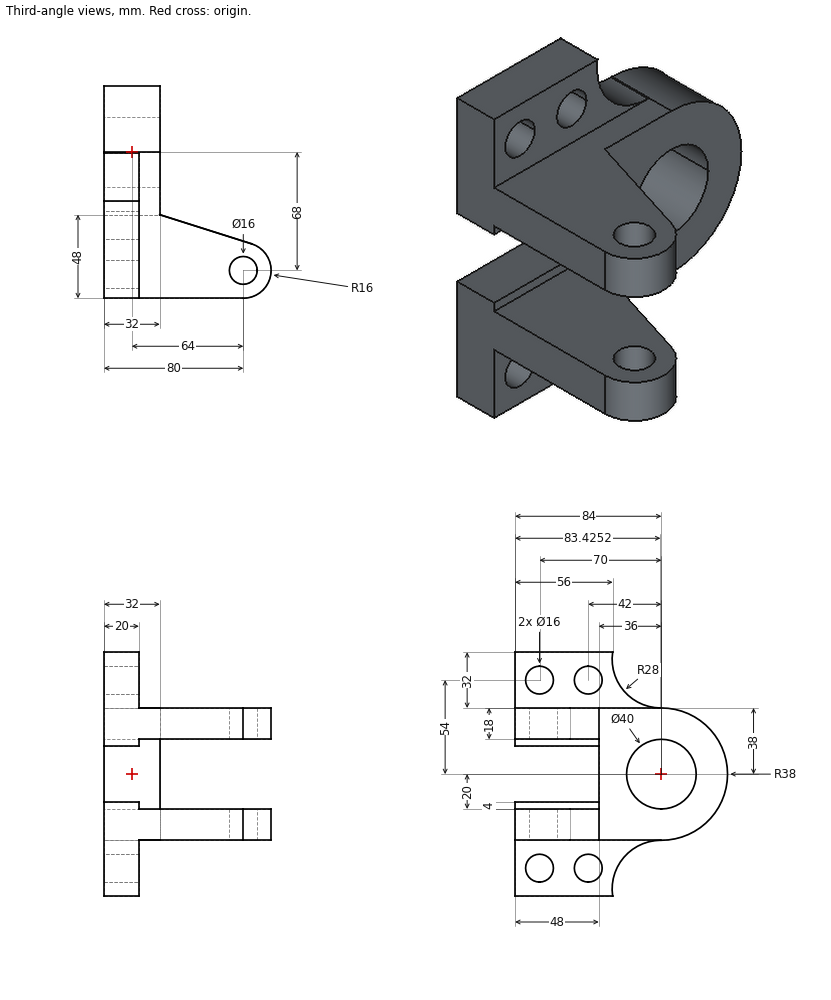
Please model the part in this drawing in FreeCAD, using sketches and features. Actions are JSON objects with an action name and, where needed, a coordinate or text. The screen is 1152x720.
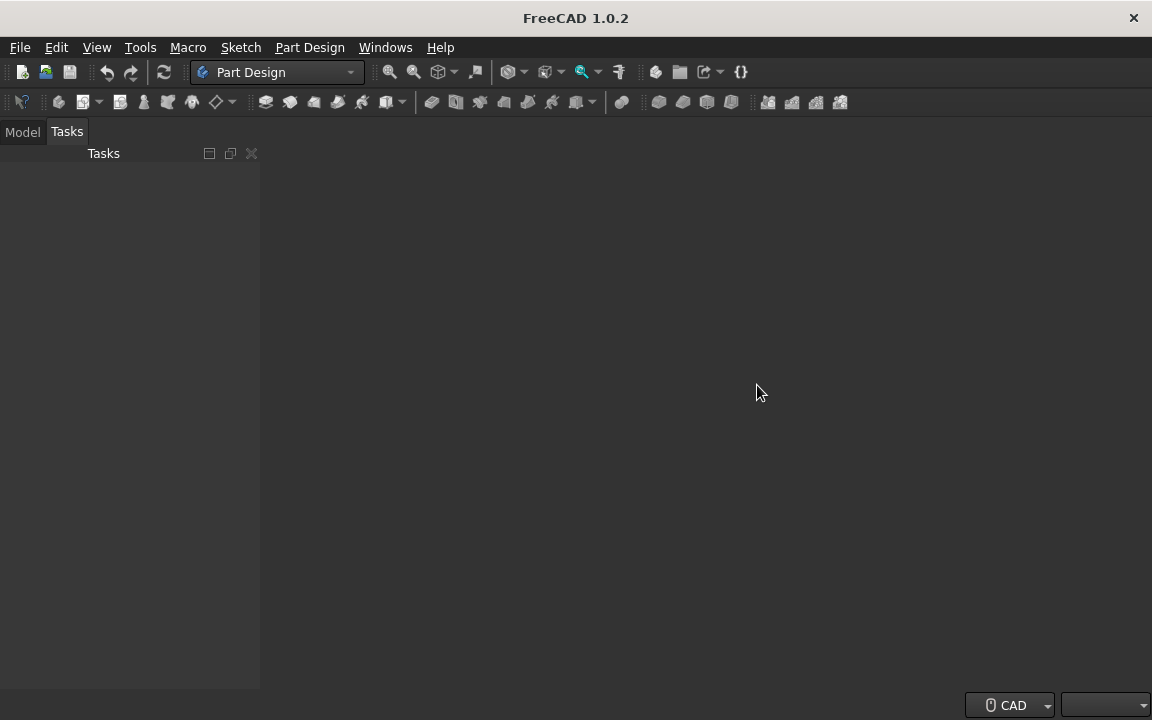
{"action": "left_click", "coordinate": [22, 72]}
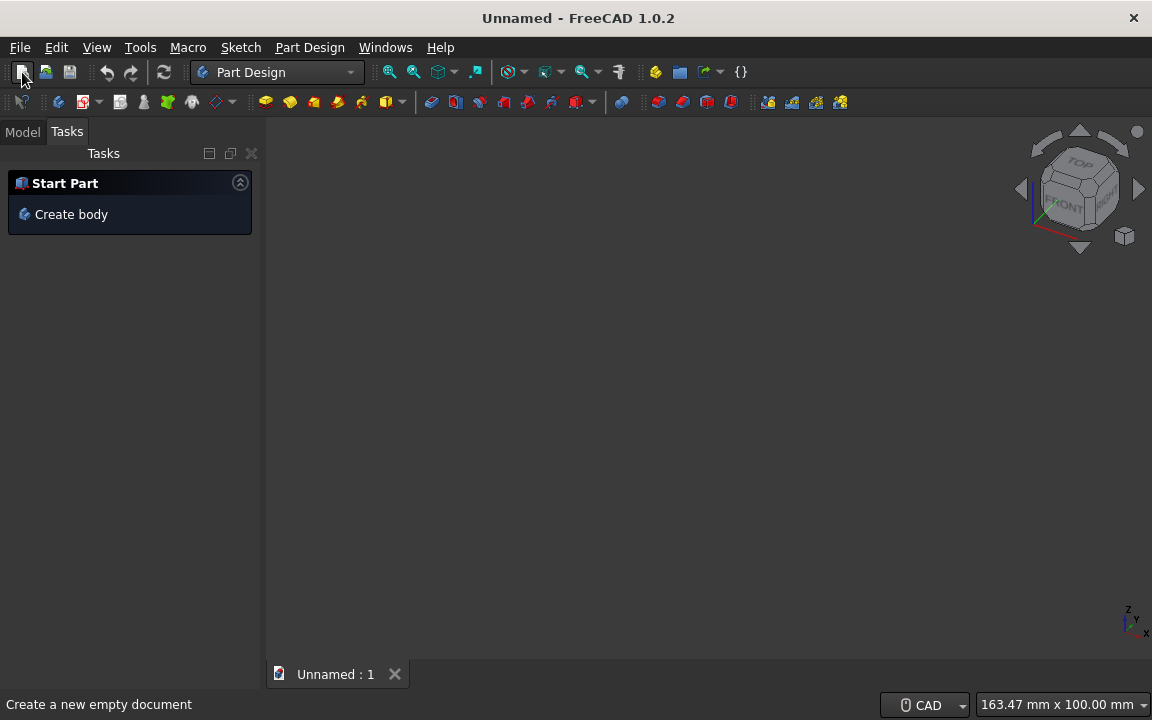
{"action": "left_click", "coordinate": [84, 102]}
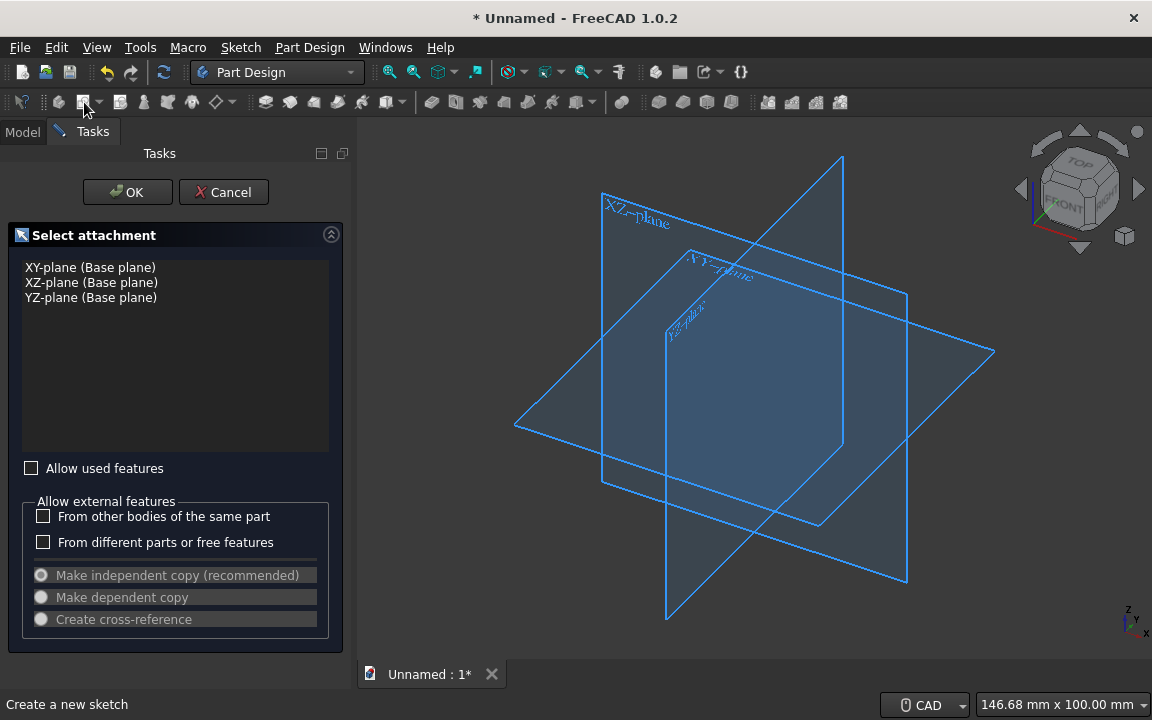
{"action": "left_click", "coordinate": [82, 298]}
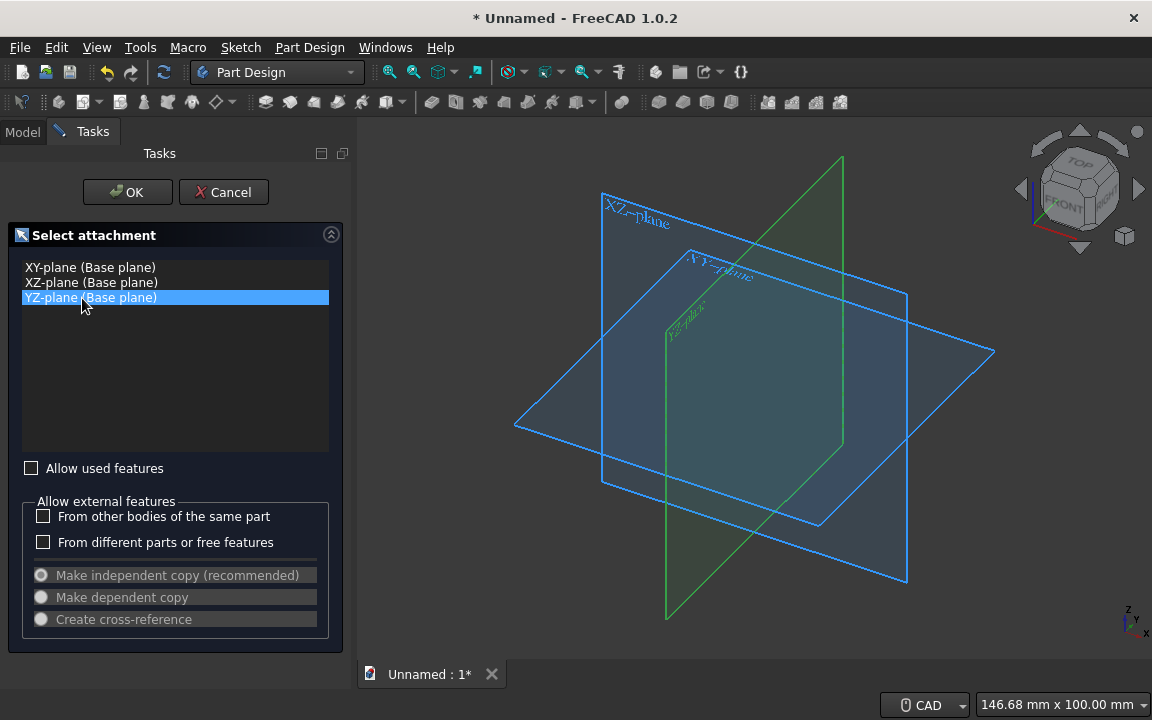
{"action": "left_click", "coordinate": [128, 192]}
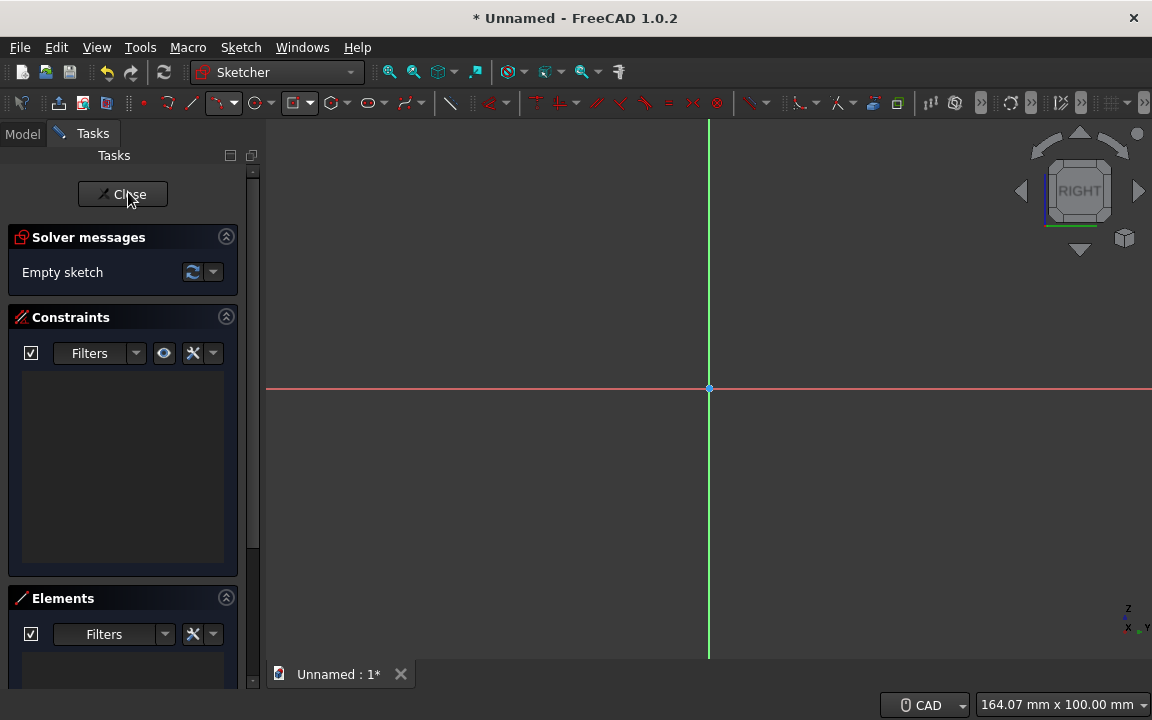
{"action": "left_click", "coordinate": [168, 104]}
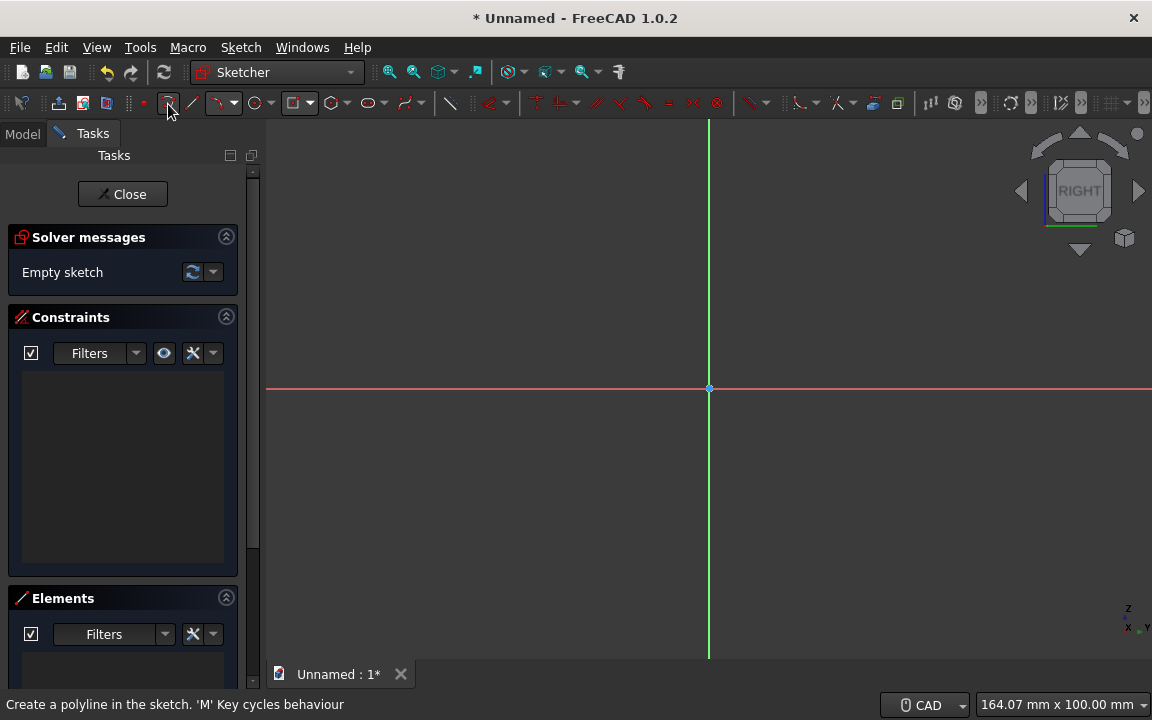
{"action": "left_click", "coordinate": [709, 184]}
{"action": "left_click", "coordinate": [515, 184]}
{"action": "left_click", "coordinate": [515, 594]}
{"action": "left_click", "coordinate": [709, 594]}
{"action": "right_click", "coordinate": [709, 594]}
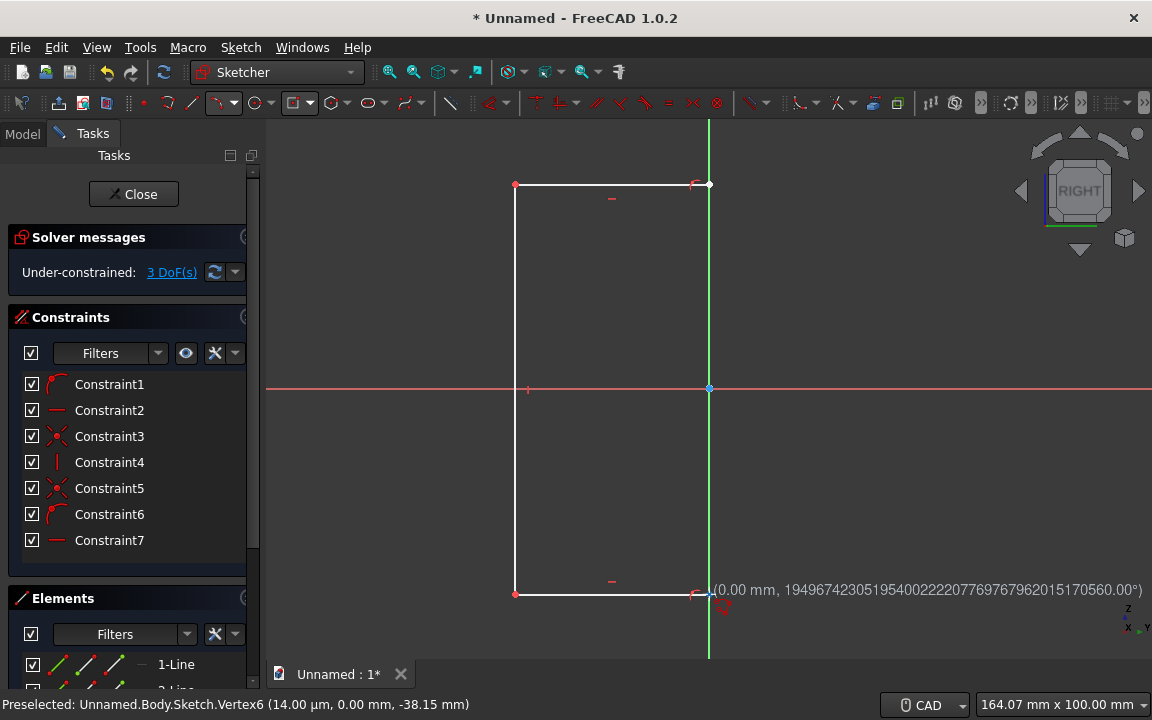
{"action": "left_click", "coordinate": [218, 104]}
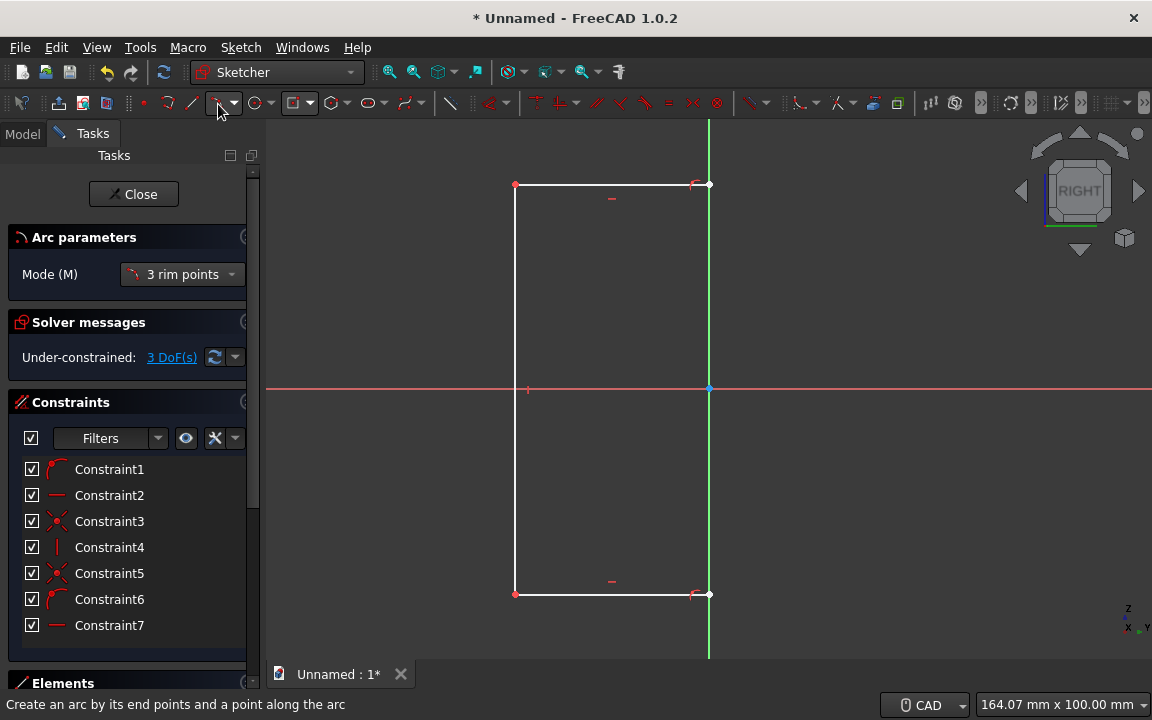
{"action": "left_click", "coordinate": [709, 595]}
{"action": "left_click", "coordinate": [709, 185]}
{"action": "left_click", "coordinate": [904, 452]}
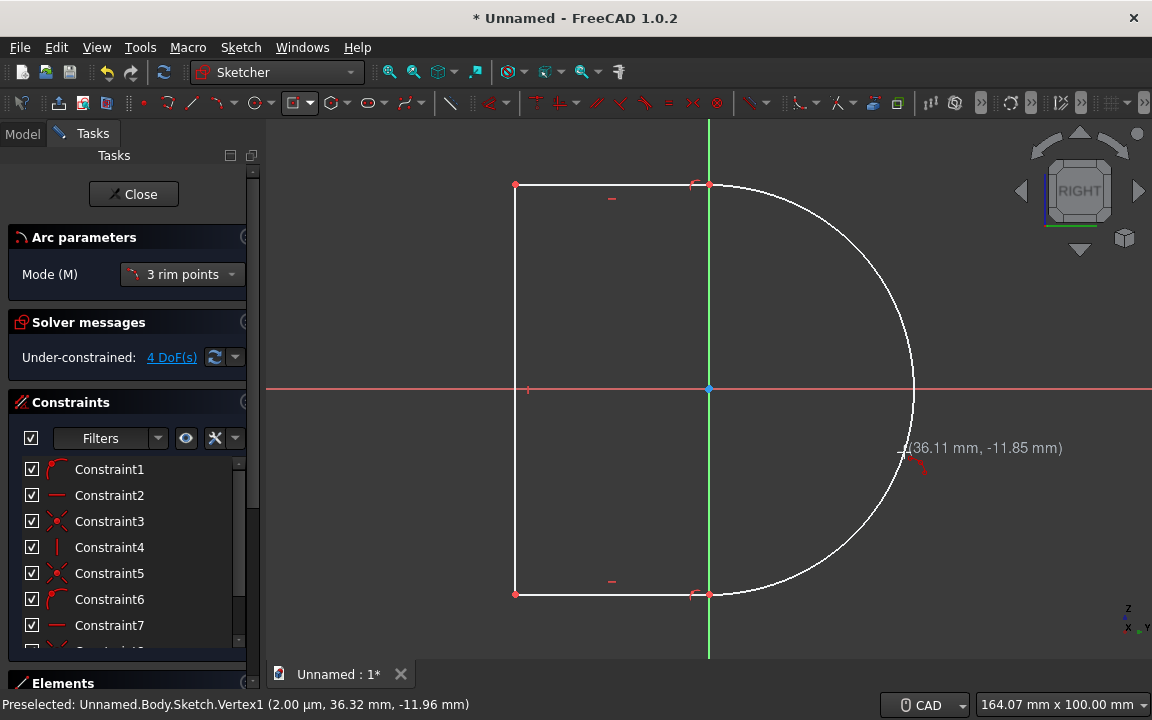
{"action": "key", "text": "g c"}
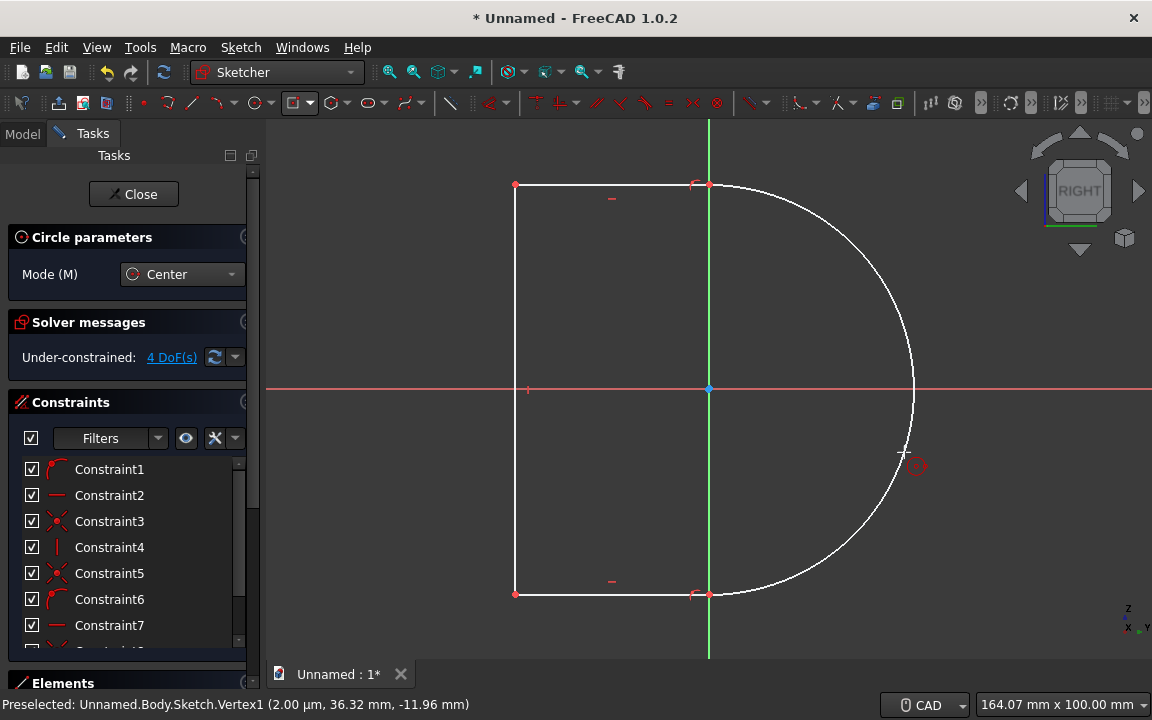
{"action": "left_click", "coordinate": [709, 389]}
{"action": "left_click", "coordinate": [785, 313]}
{"action": "key", "text": "Escape"}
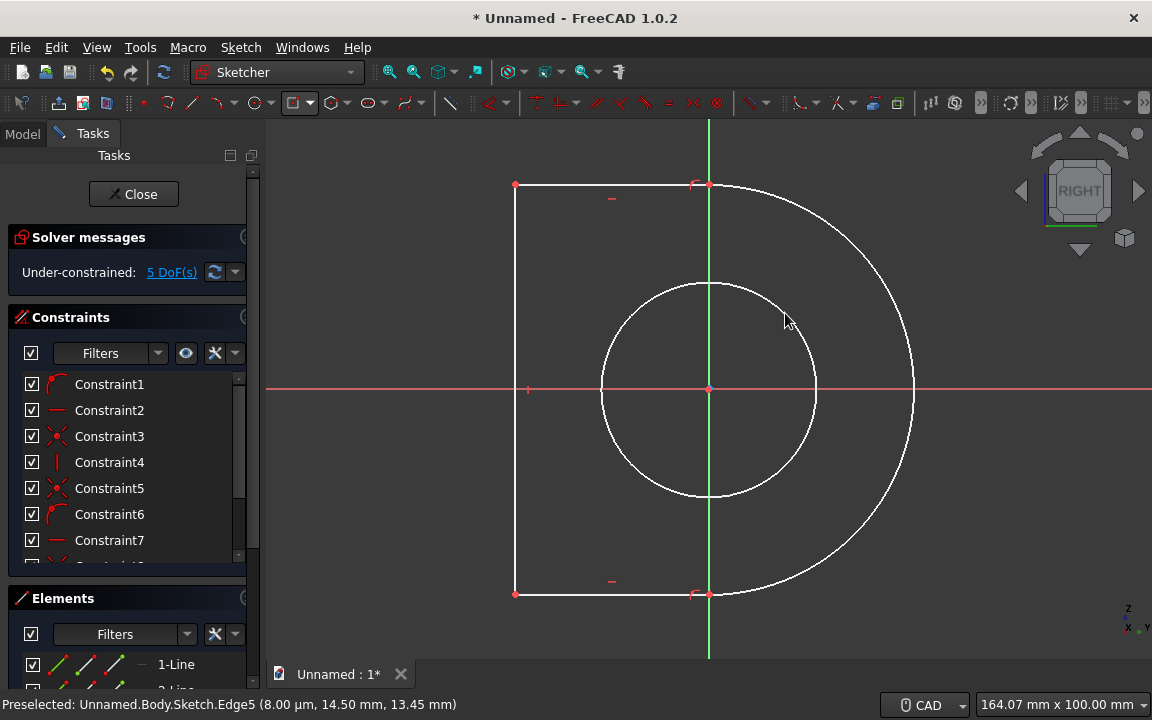
{"action": "left_click_drag", "start_coordinate": [699, 379], "coordinate": [719, 400]}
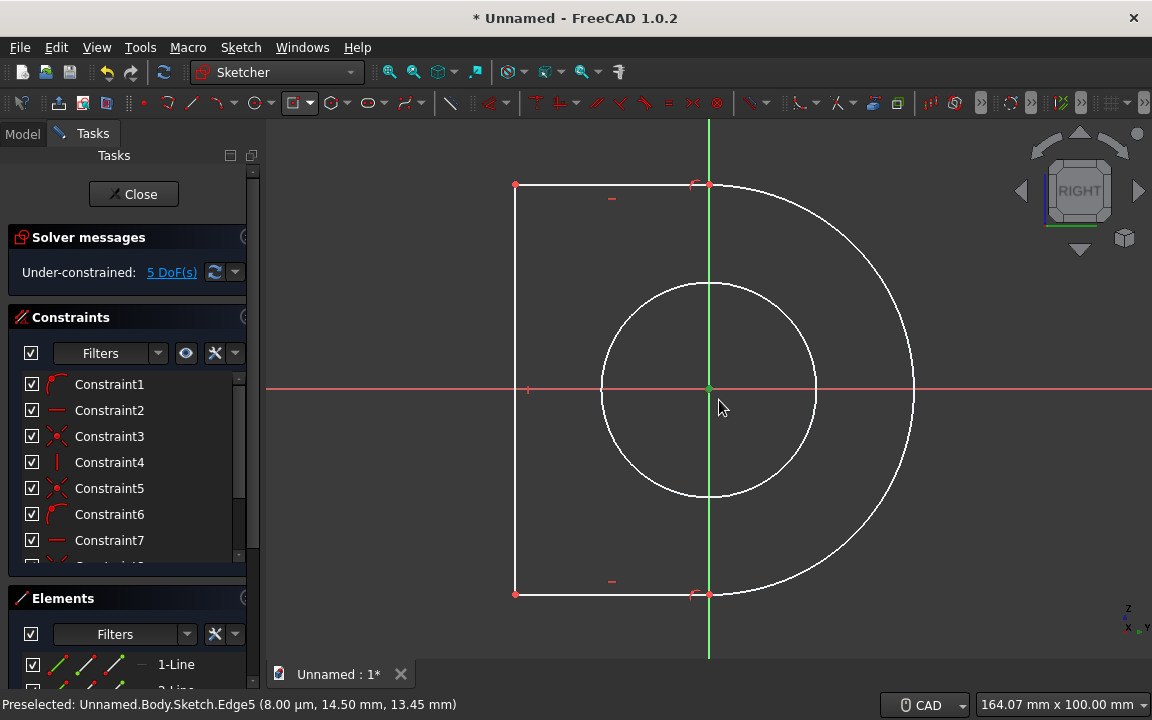
{"action": "left_click", "coordinate": [536, 104]}